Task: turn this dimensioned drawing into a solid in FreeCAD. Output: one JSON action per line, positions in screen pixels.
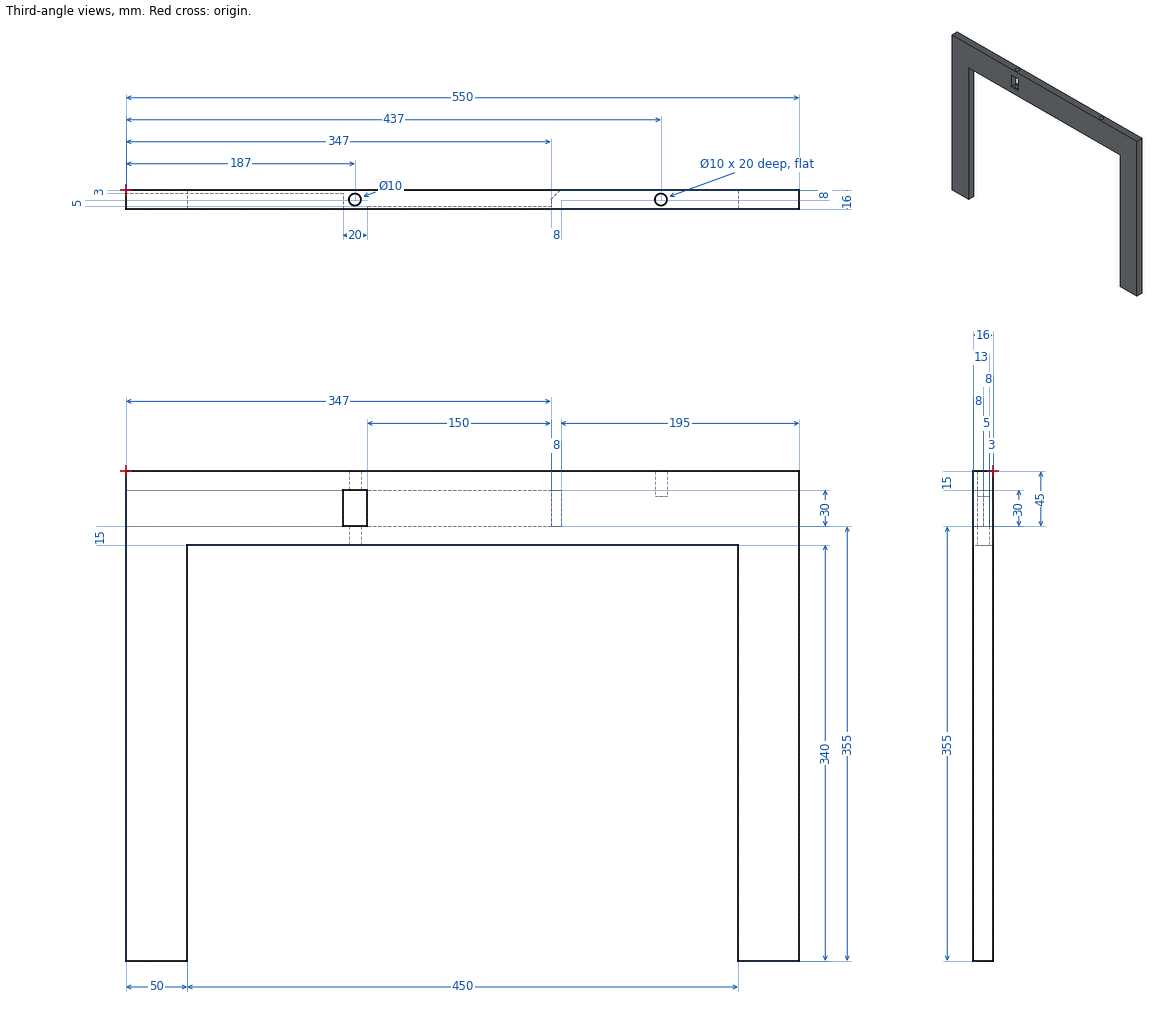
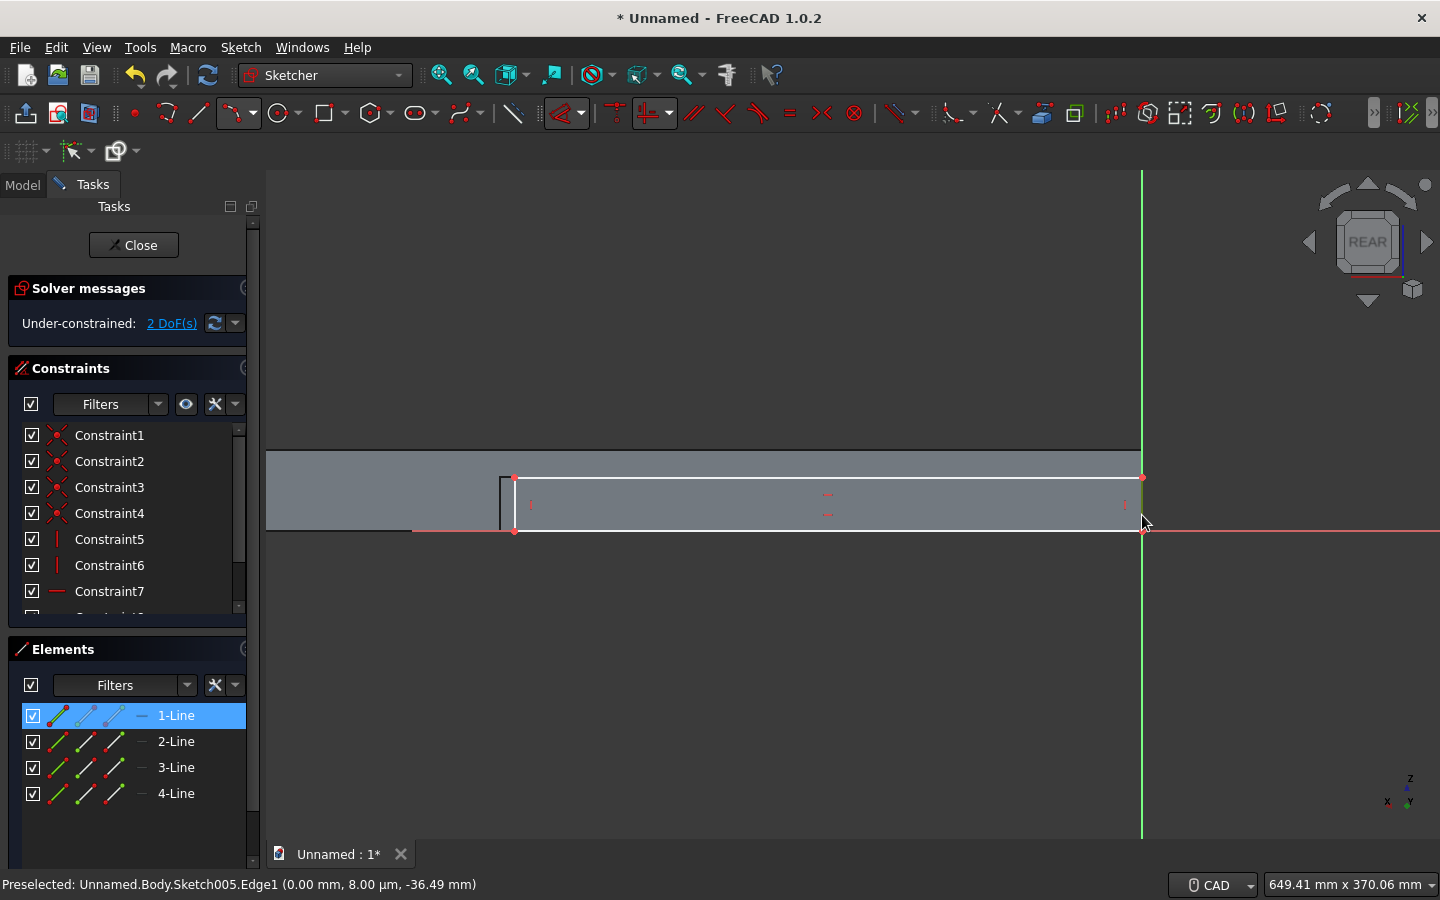
{"action": "left_click", "coordinate": [584, 114]}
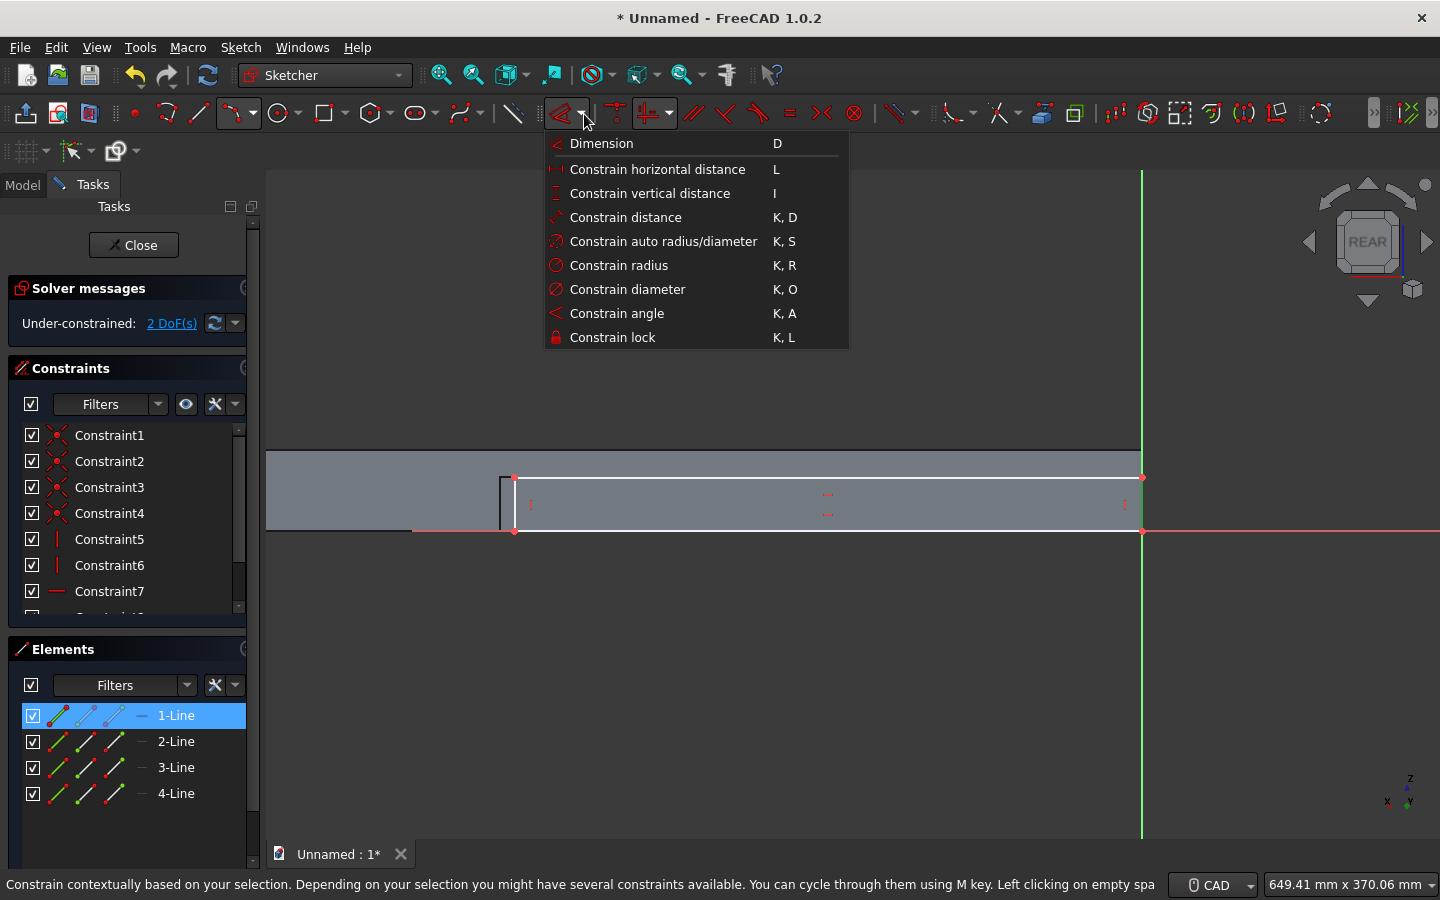
{"action": "left_click", "coordinate": [697, 193]}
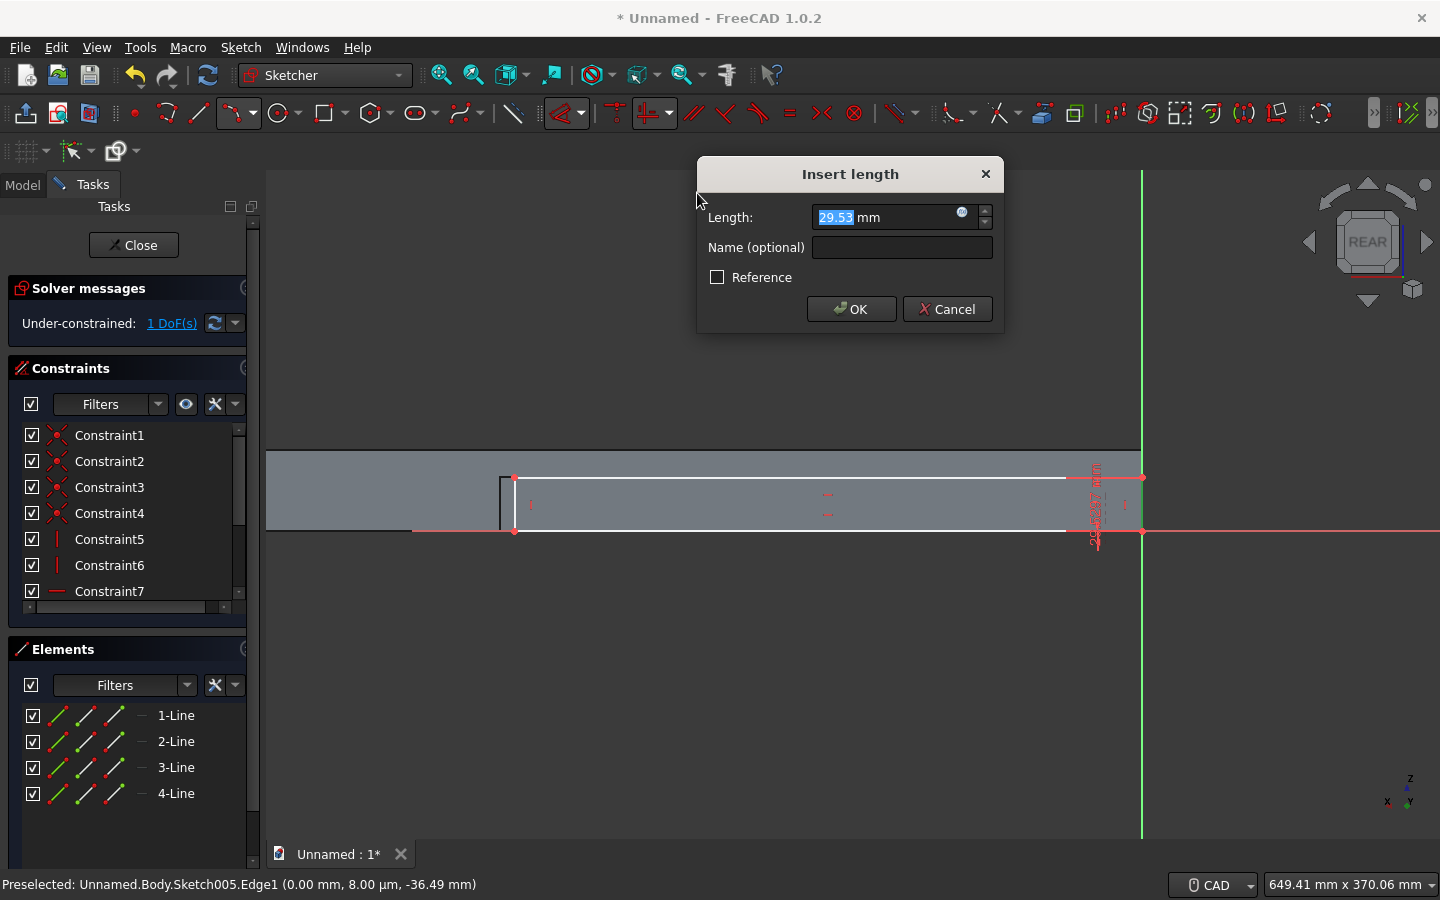
{"action": "type", "text": "30"}
{"action": "key", "text": "Return"}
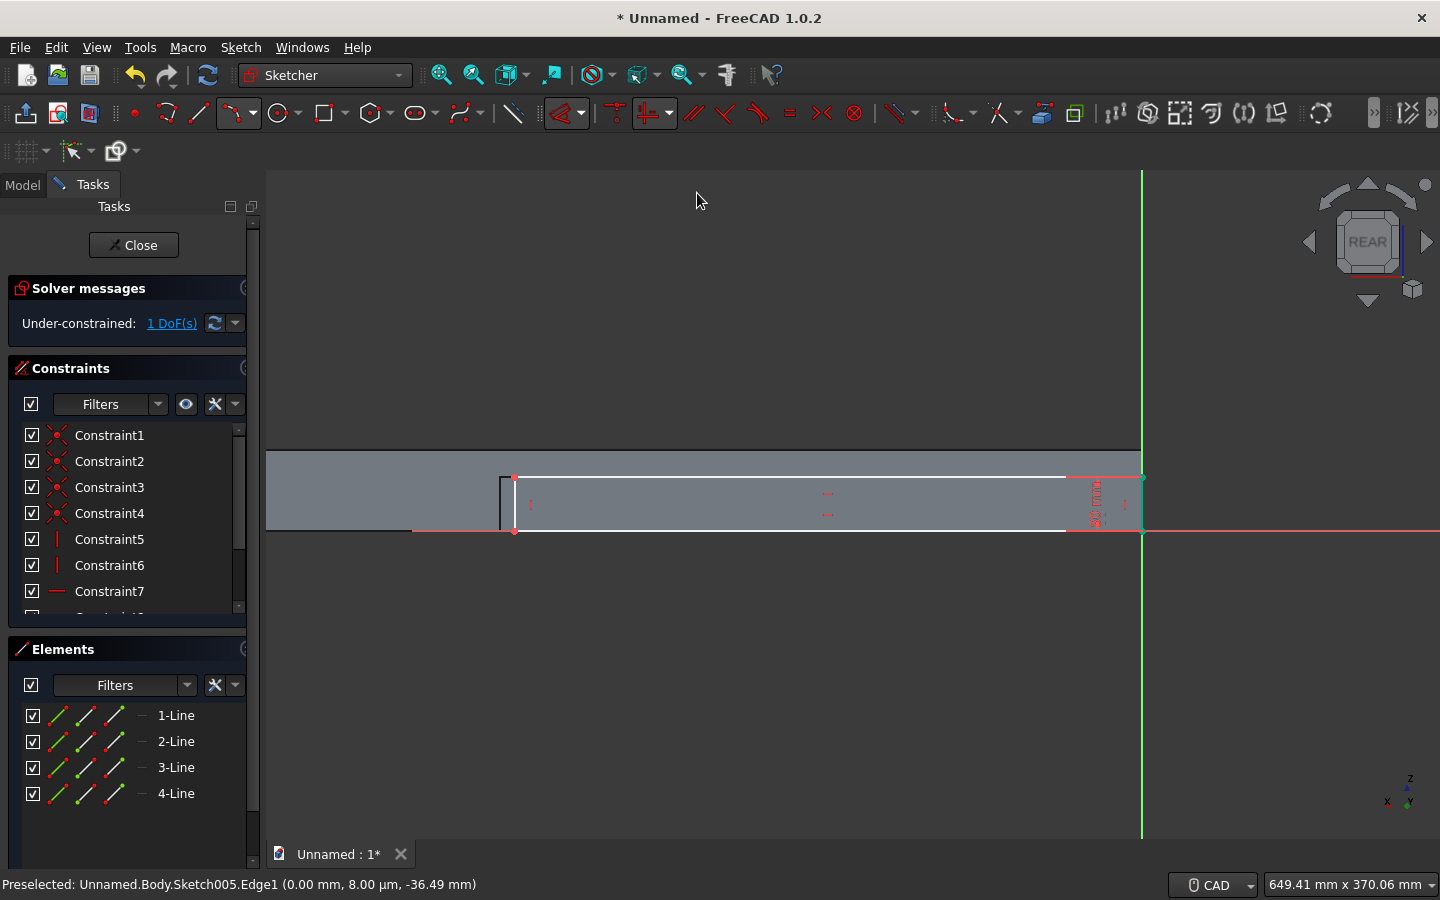
{"action": "left_click", "coordinate": [954, 477]}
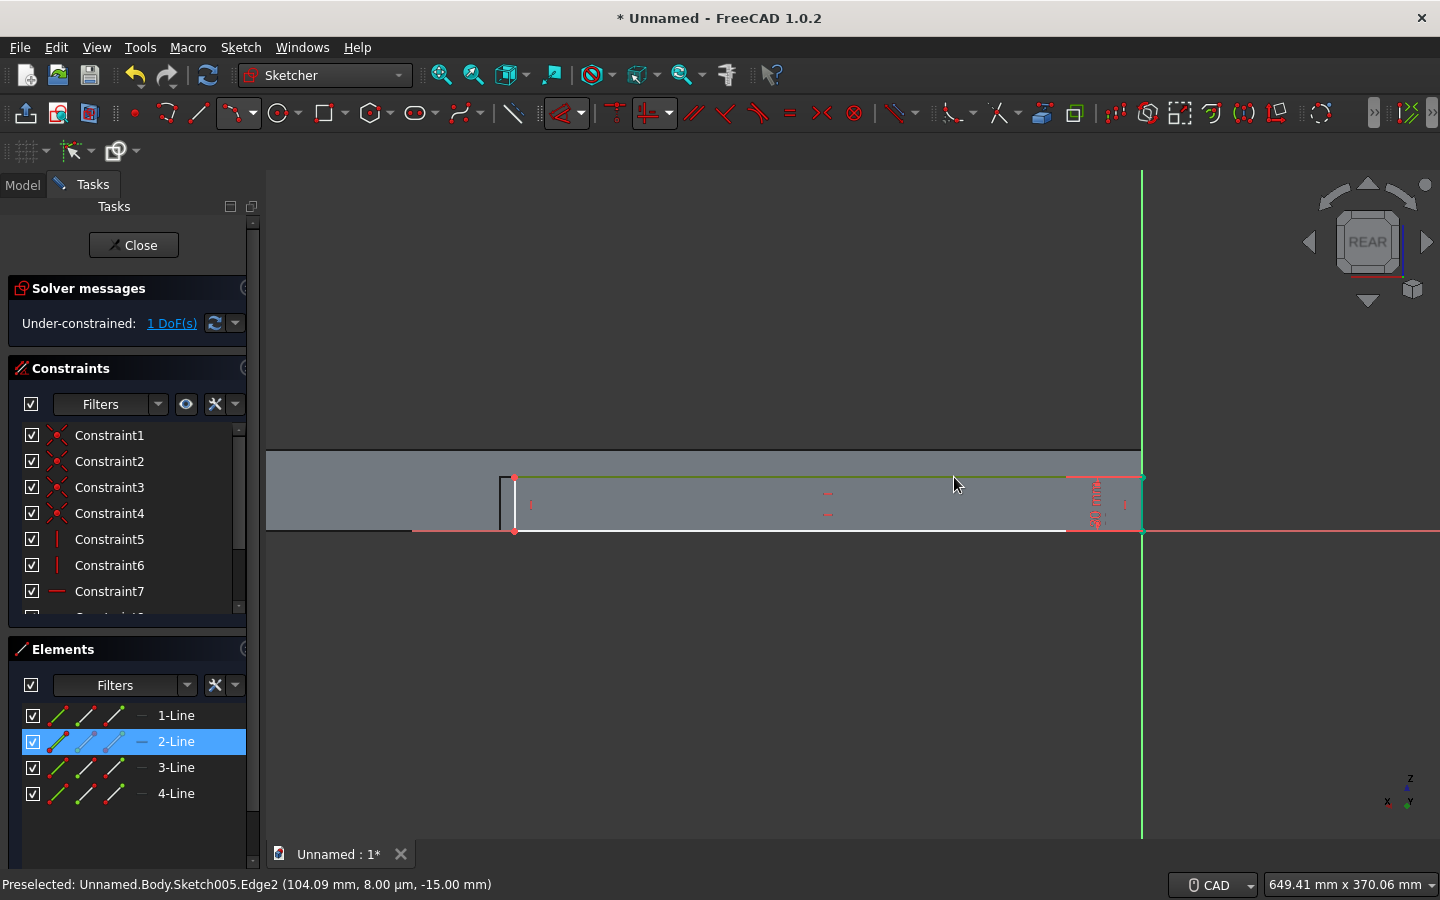
{"action": "key", "text": "l"}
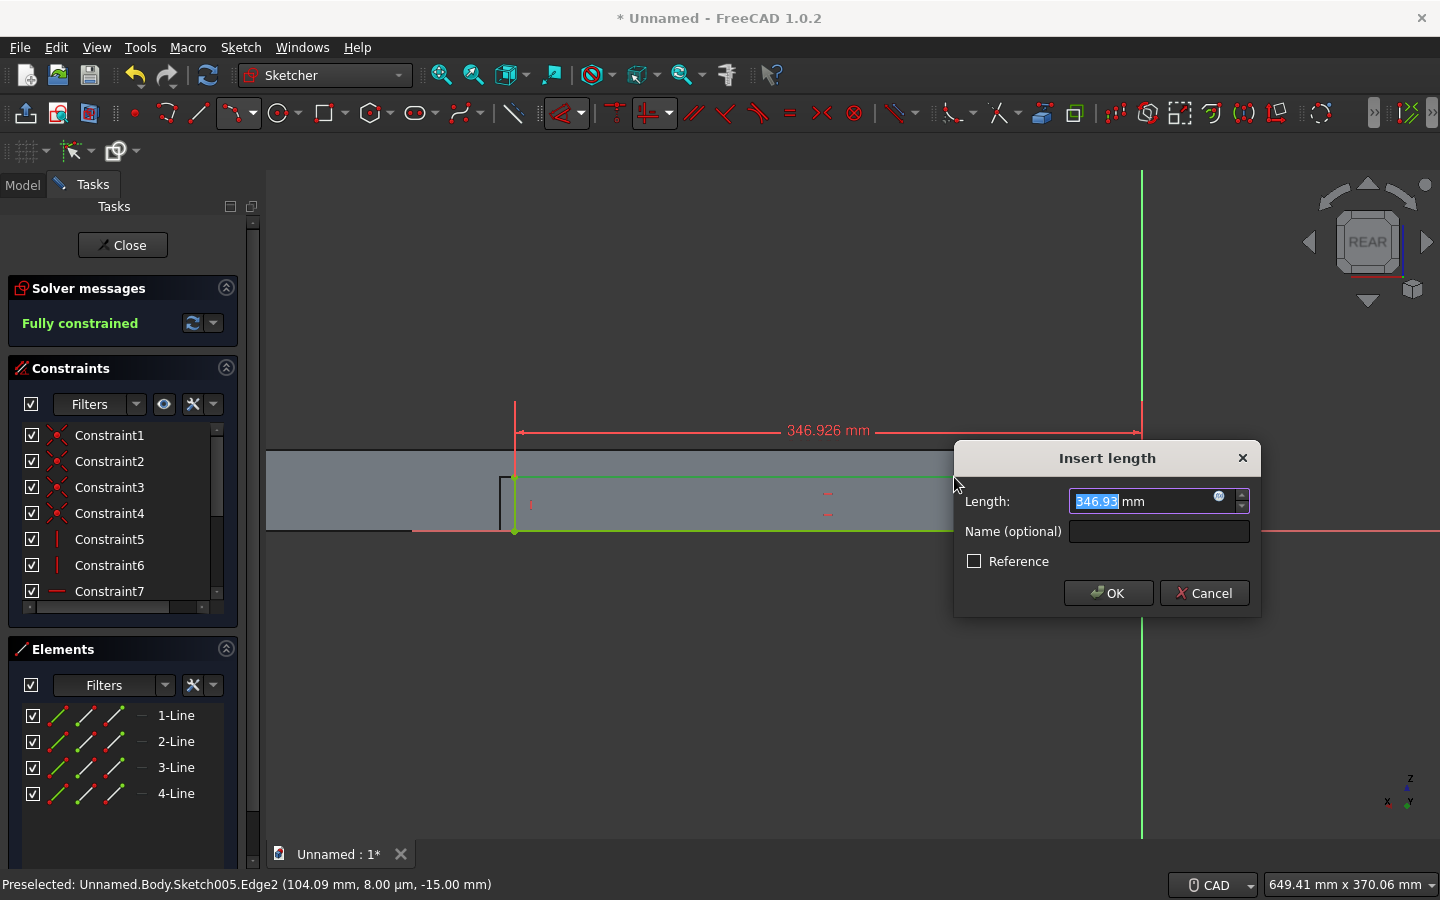
{"action": "type", "text": "347"}
{"action": "key", "text": "Return"}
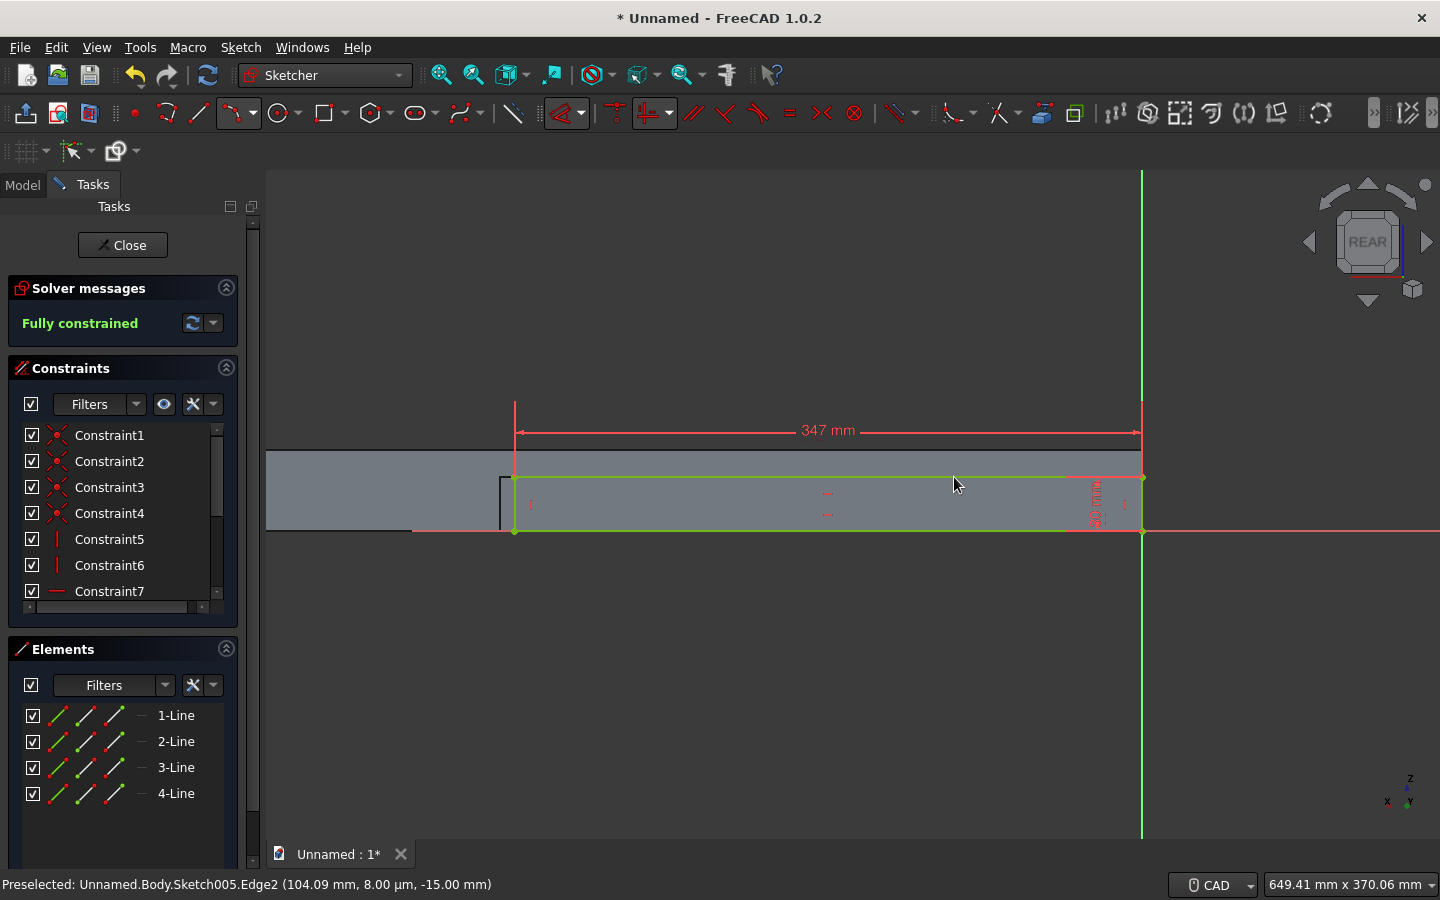
{"action": "left_click", "coordinate": [123, 245]}